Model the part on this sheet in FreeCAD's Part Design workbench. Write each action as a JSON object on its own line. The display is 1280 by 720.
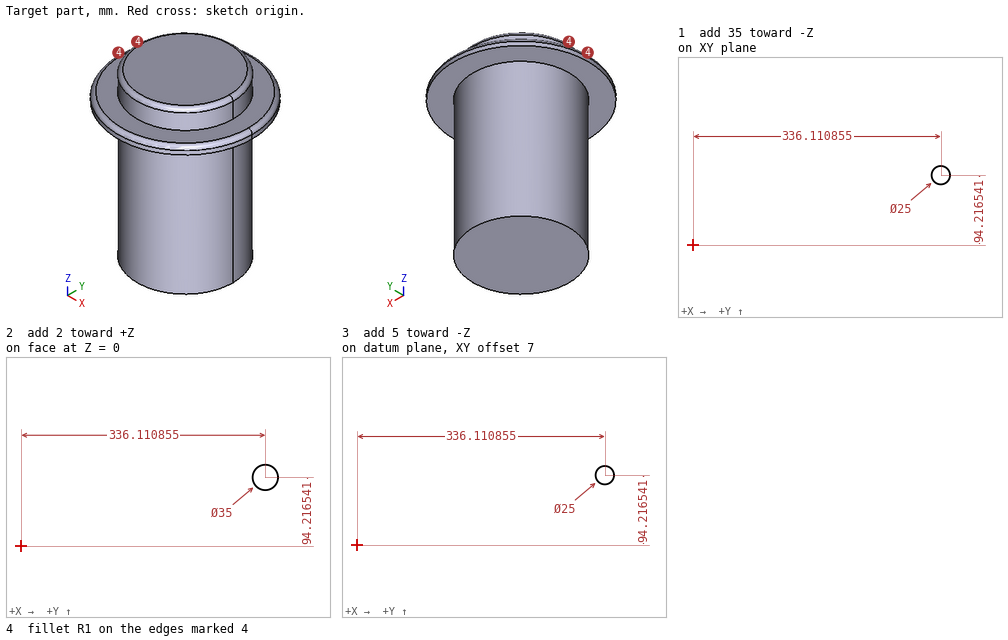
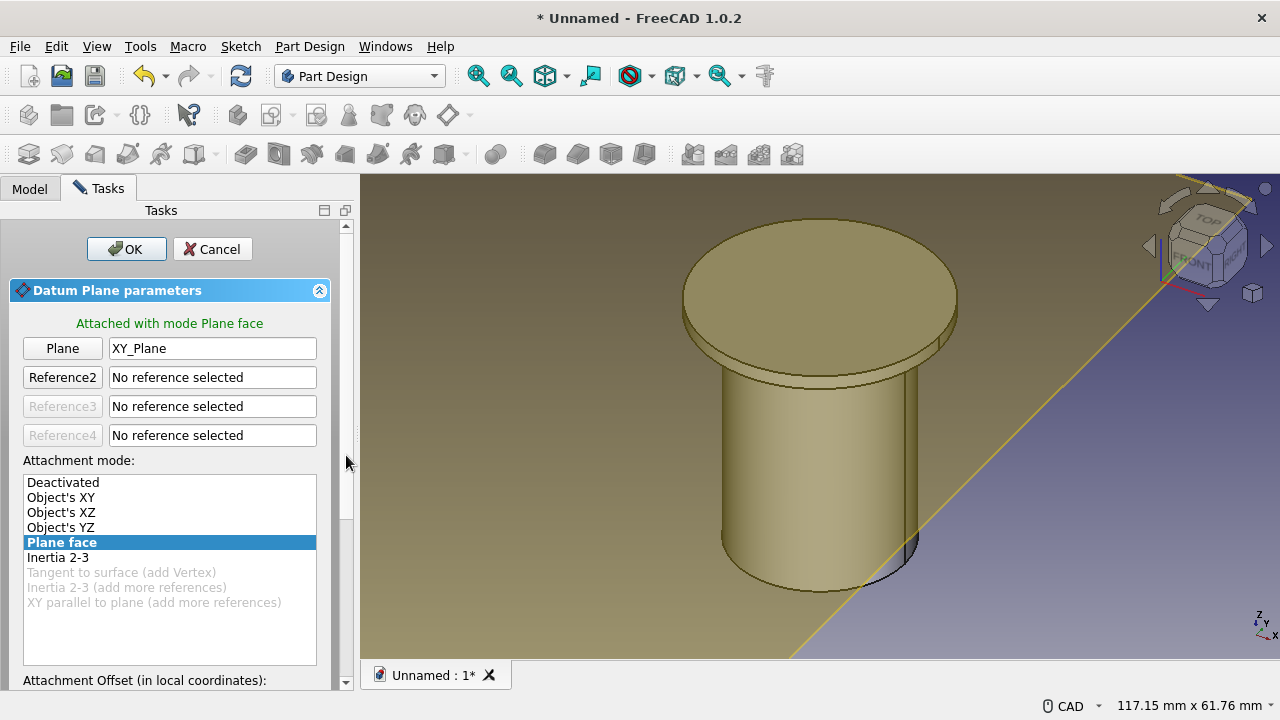
{"action": "left_click", "coordinate": [127, 249]}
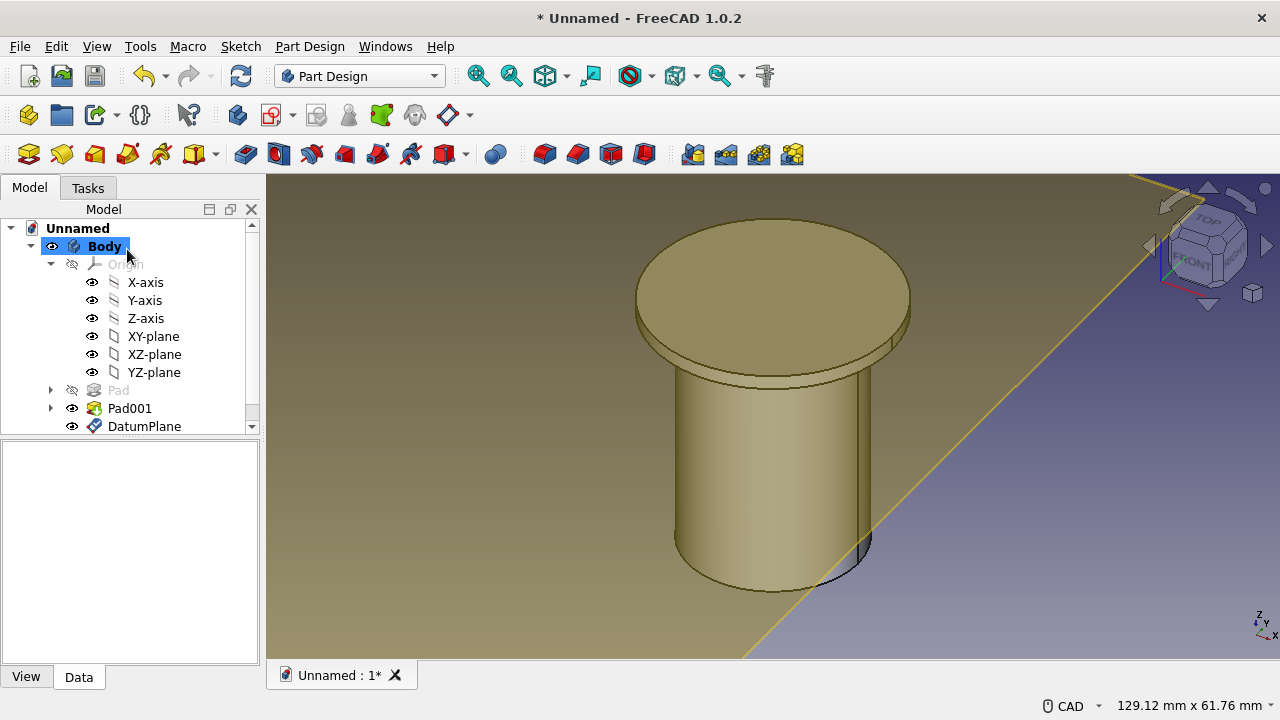
{"action": "left_click", "coordinate": [117, 426]}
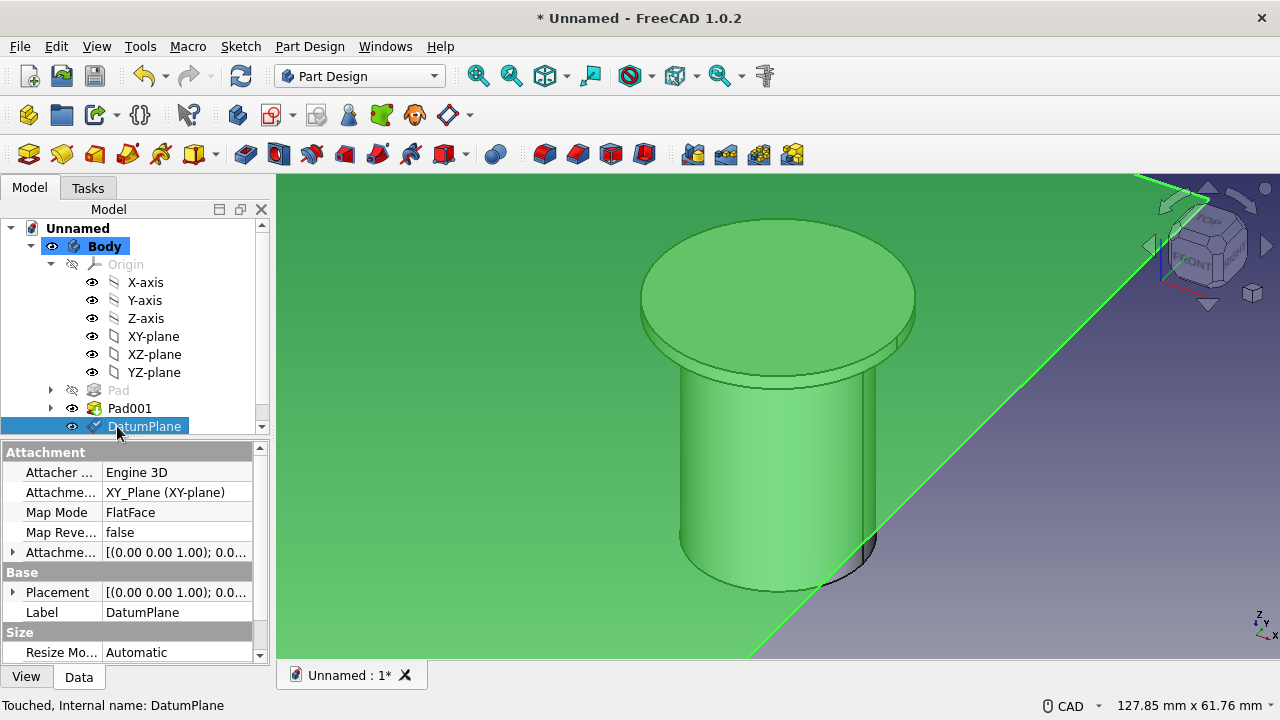
{"action": "left_click", "coordinate": [270, 116]}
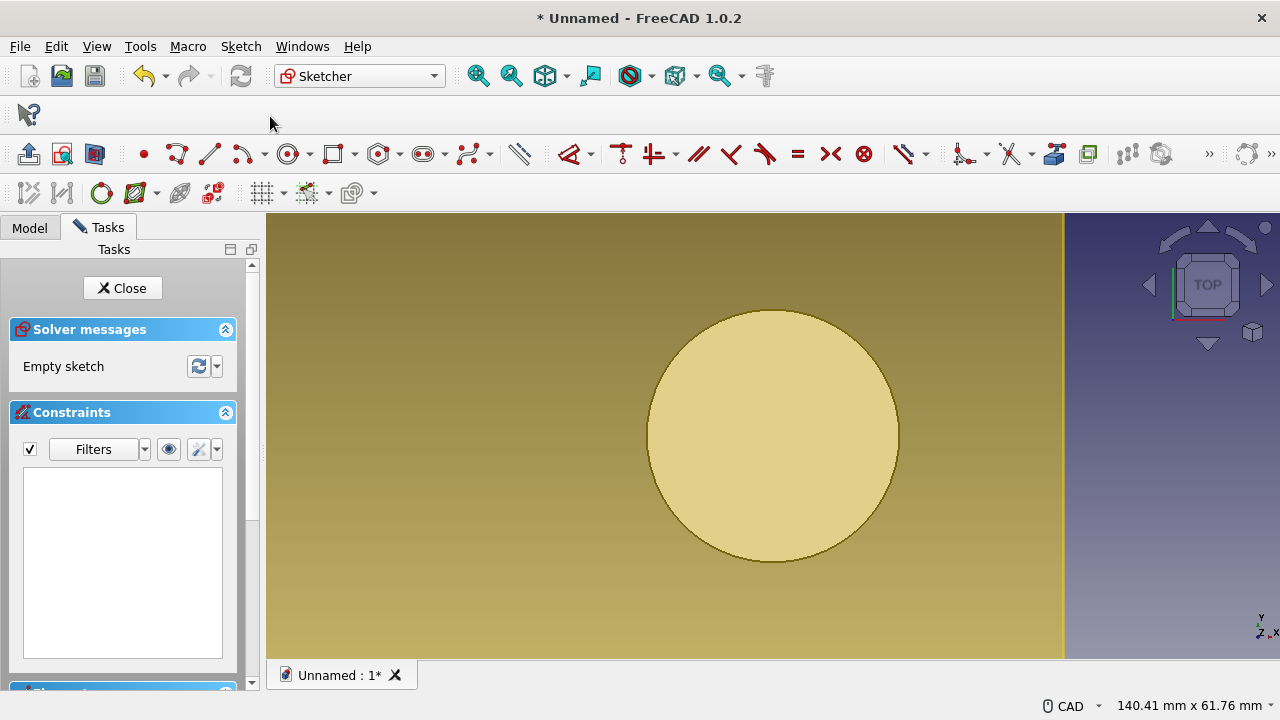
{"action": "scroll", "coordinate": [912, 436], "scroll_direction": "up", "scroll_amount": 2}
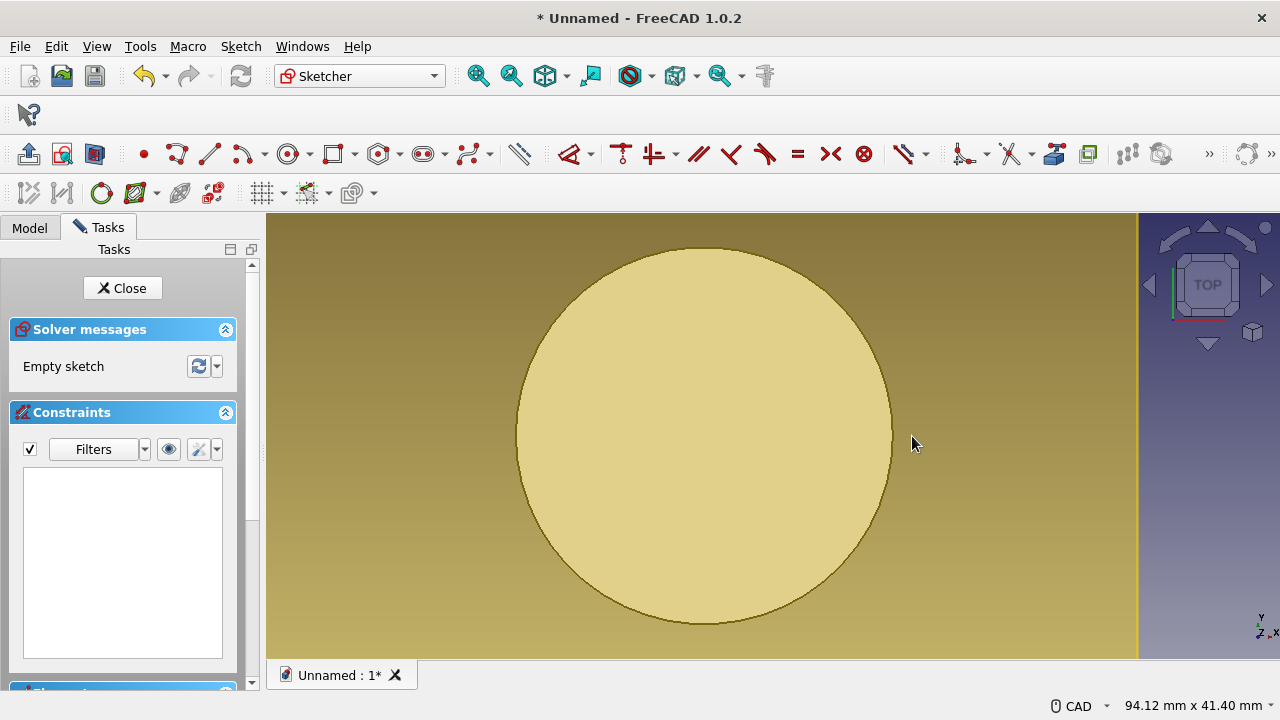
{"action": "left_click", "coordinate": [288, 154]}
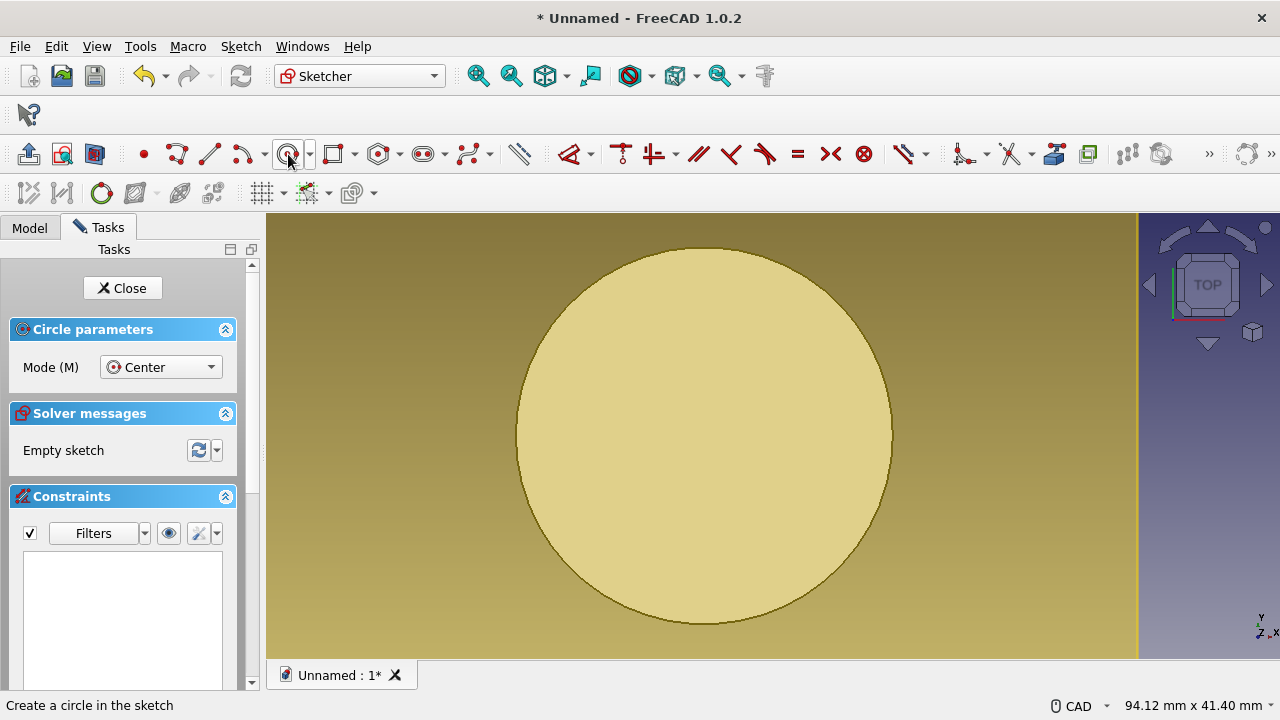
{"action": "left_click", "coordinate": [704, 436]}
{"action": "mouse_move", "coordinate": [800, 341]}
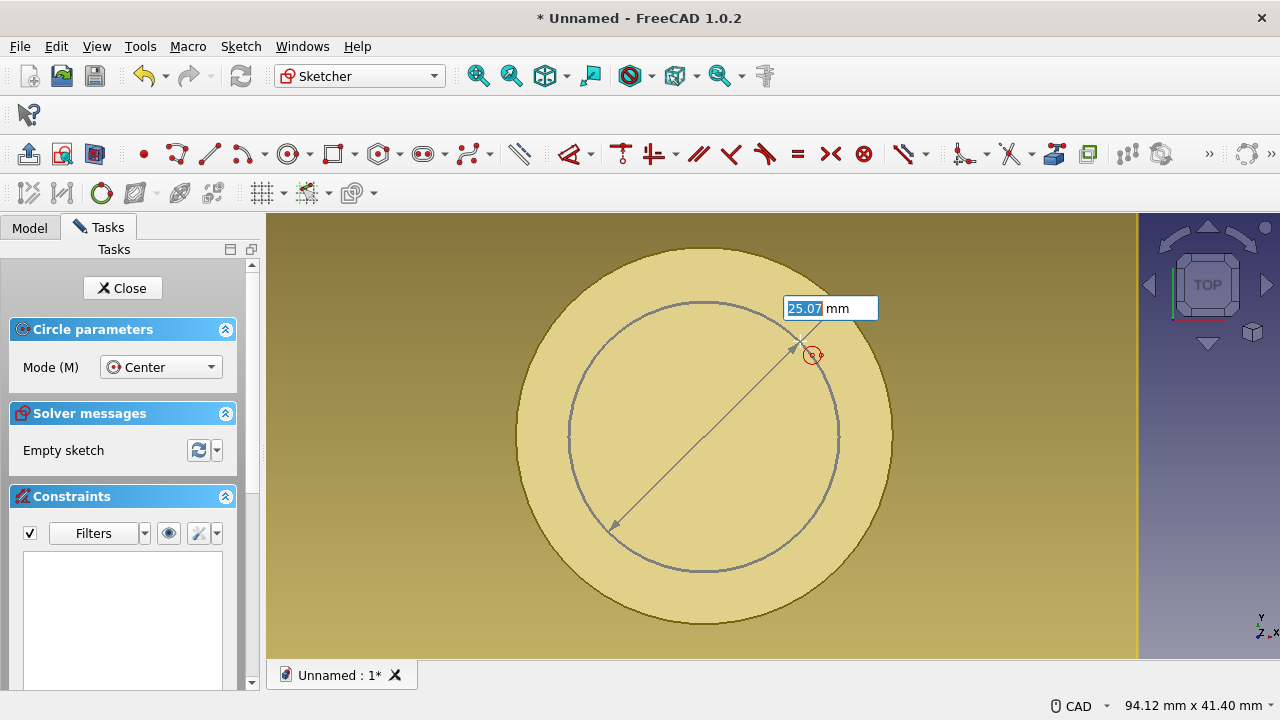
{"action": "type", "text": "25"}
{"action": "key", "text": "Return"}
{"action": "key", "text": "Escape"}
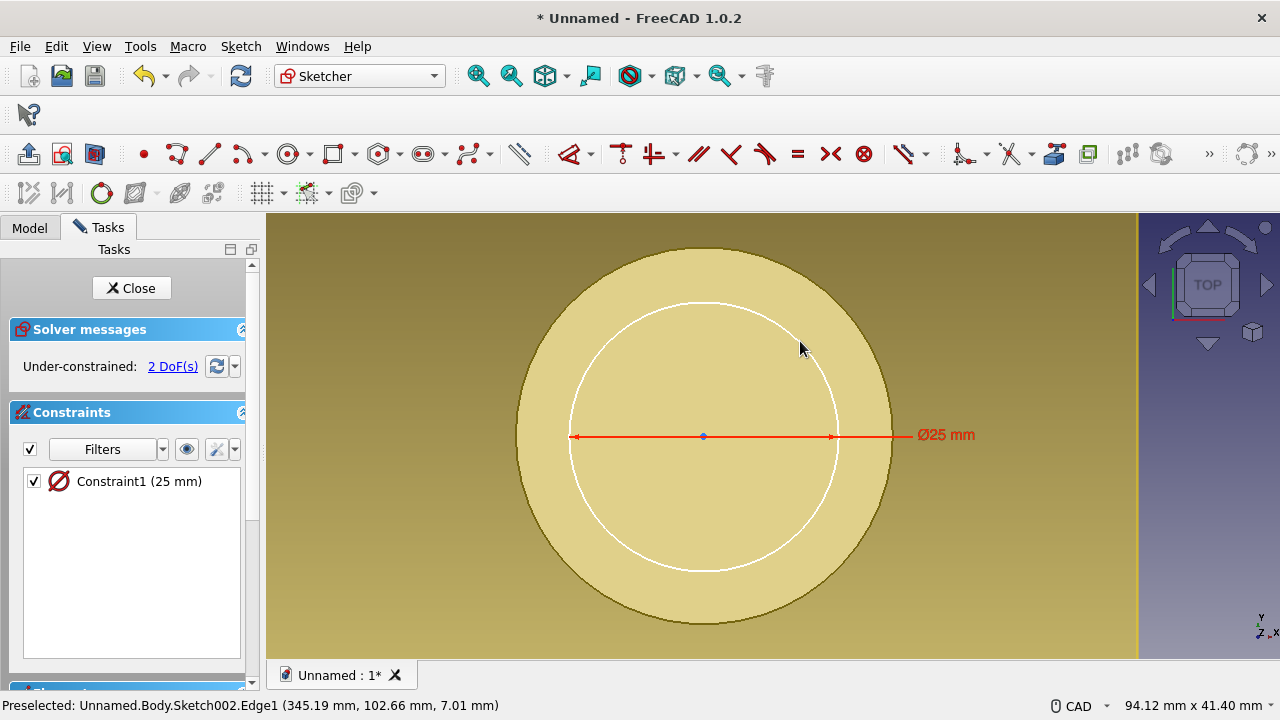
{"action": "left_click", "coordinate": [568, 154]}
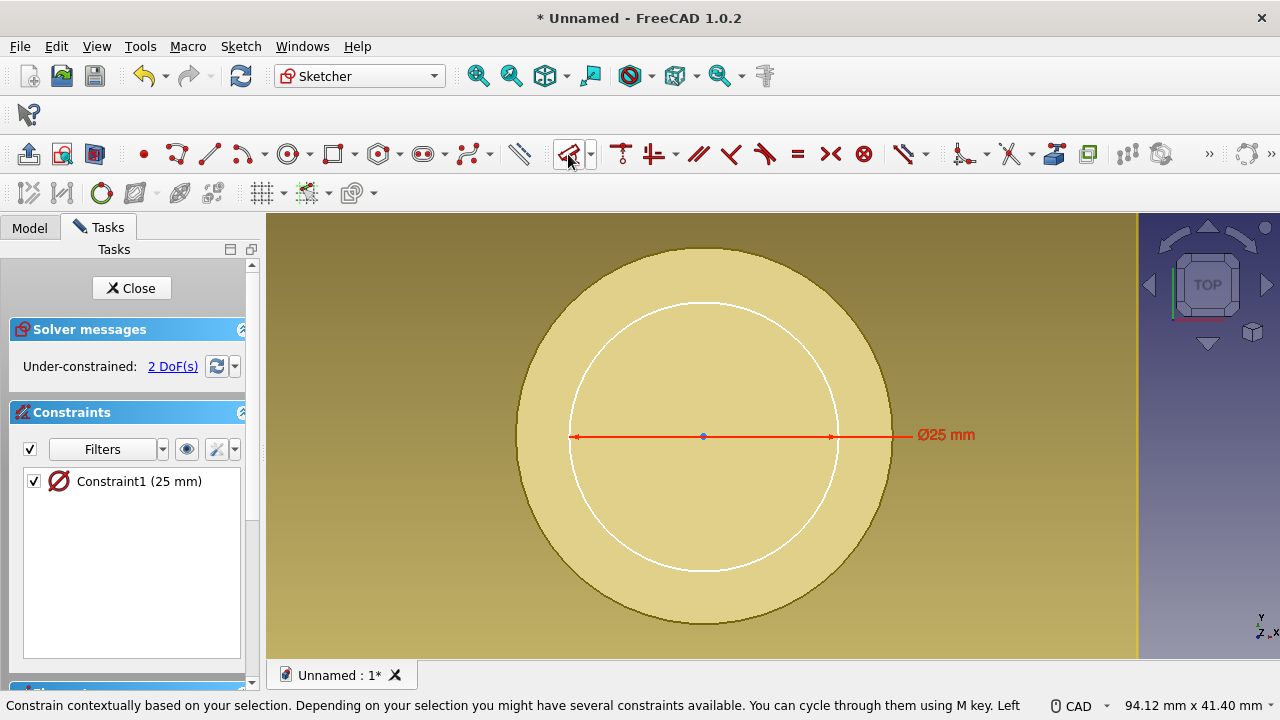
{"action": "left_click", "coordinate": [704, 437]}
{"action": "left_click", "coordinate": [738, 534]}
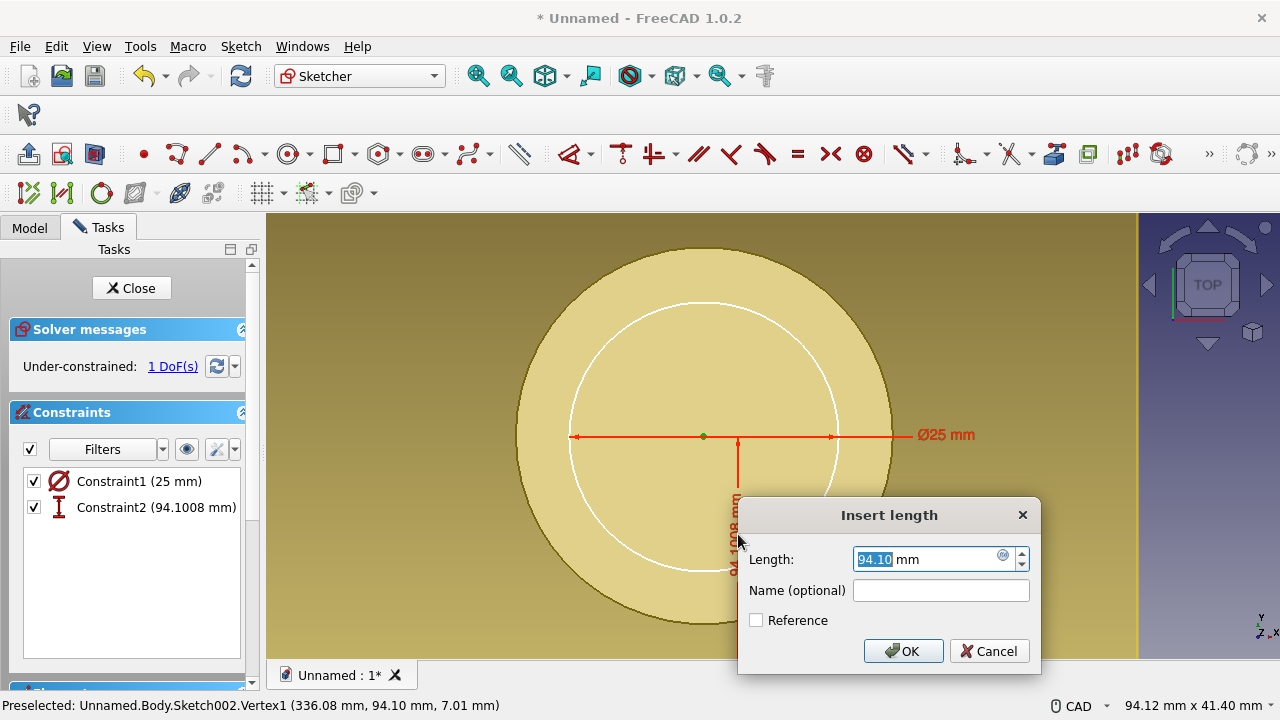
{"action": "type", "text": "94.216541"}
{"action": "key", "text": "Return"}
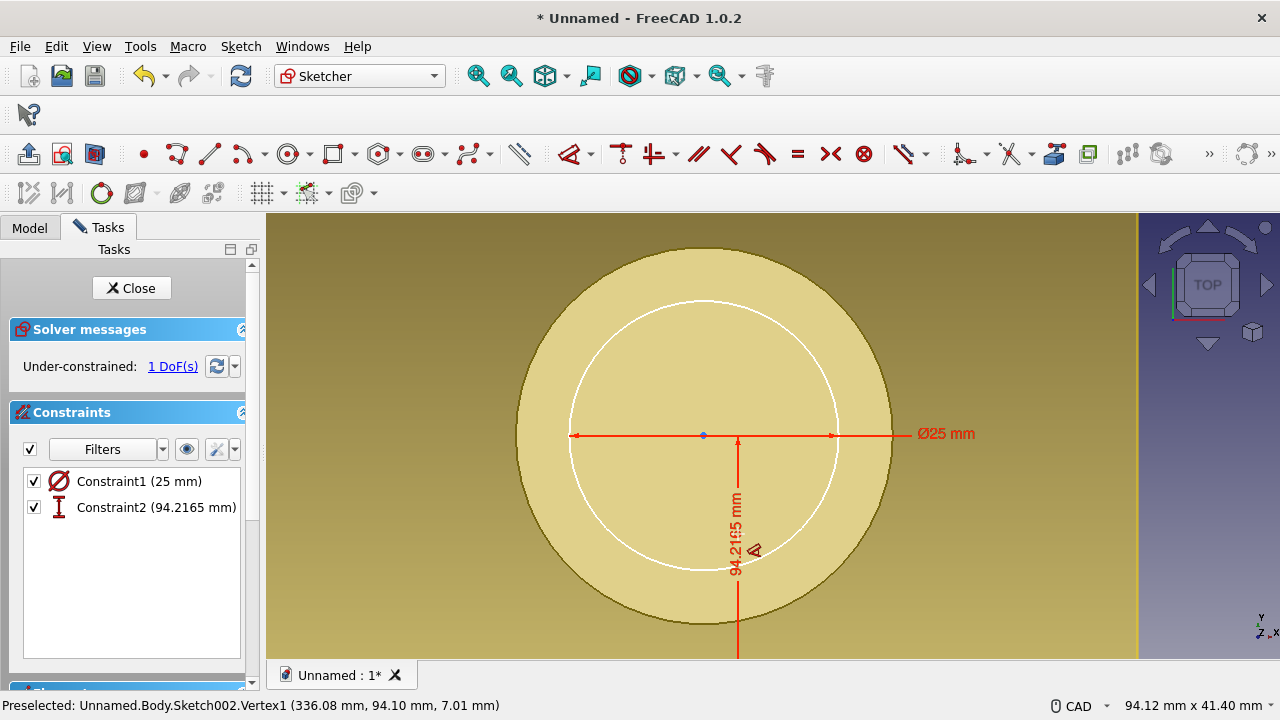
{"action": "left_click", "coordinate": [704, 436]}
{"action": "left_click", "coordinate": [499, 402]}